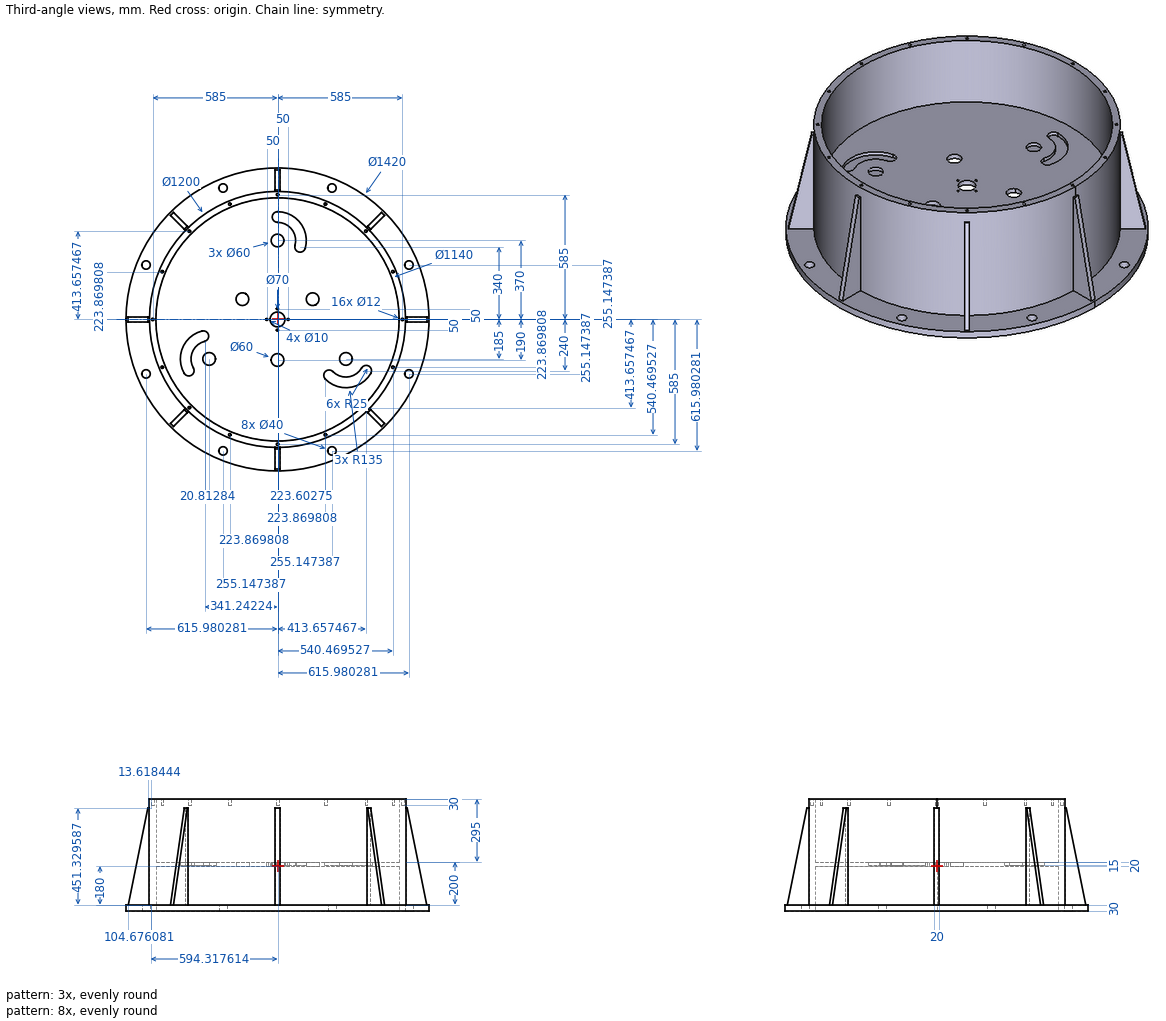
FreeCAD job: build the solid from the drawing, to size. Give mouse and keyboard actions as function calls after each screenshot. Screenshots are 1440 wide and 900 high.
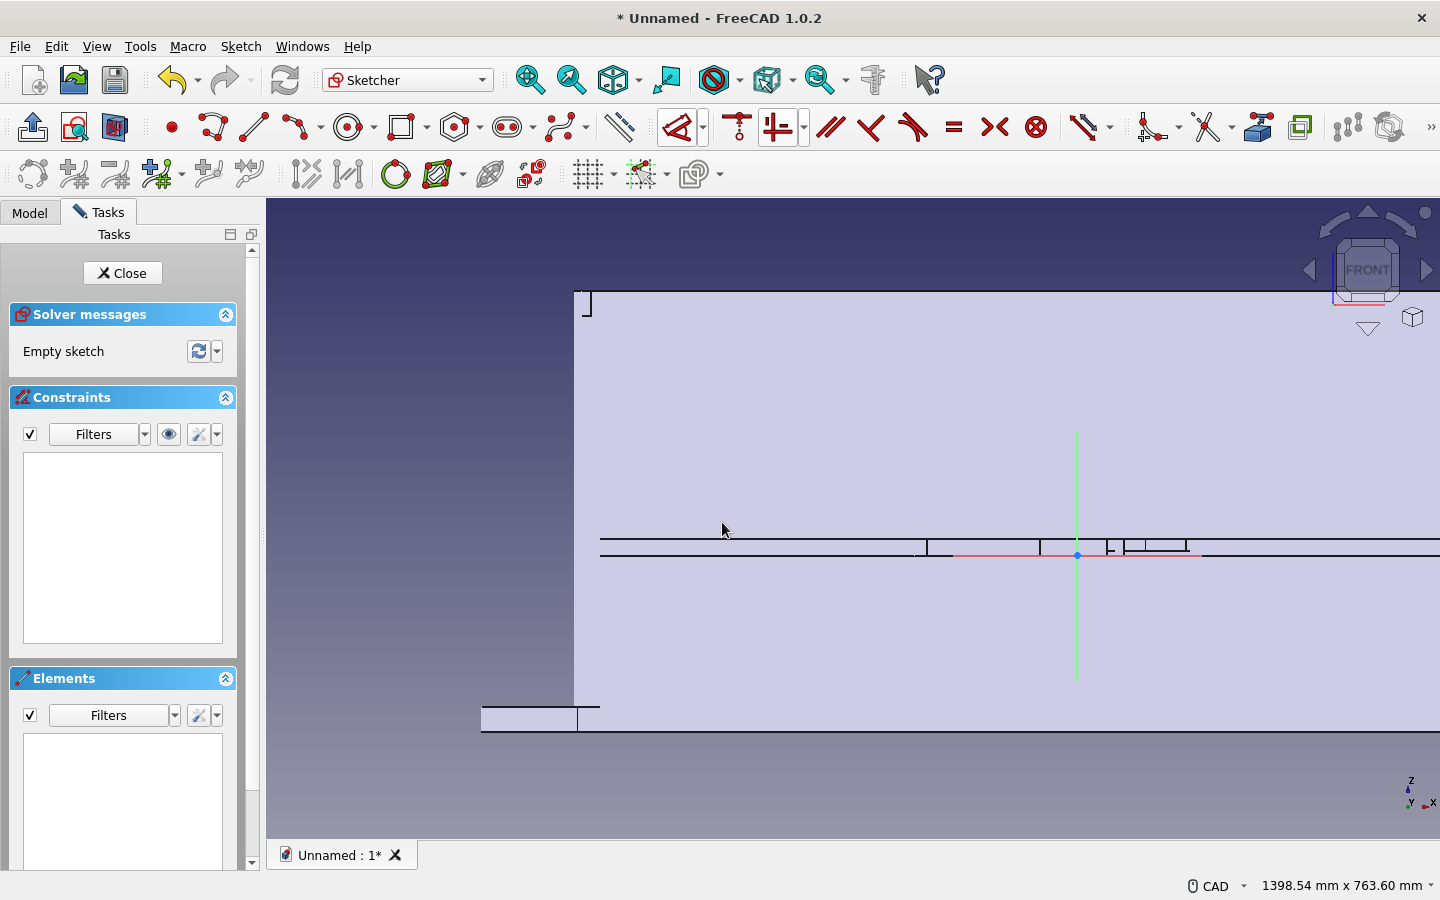
key(g)
key(m)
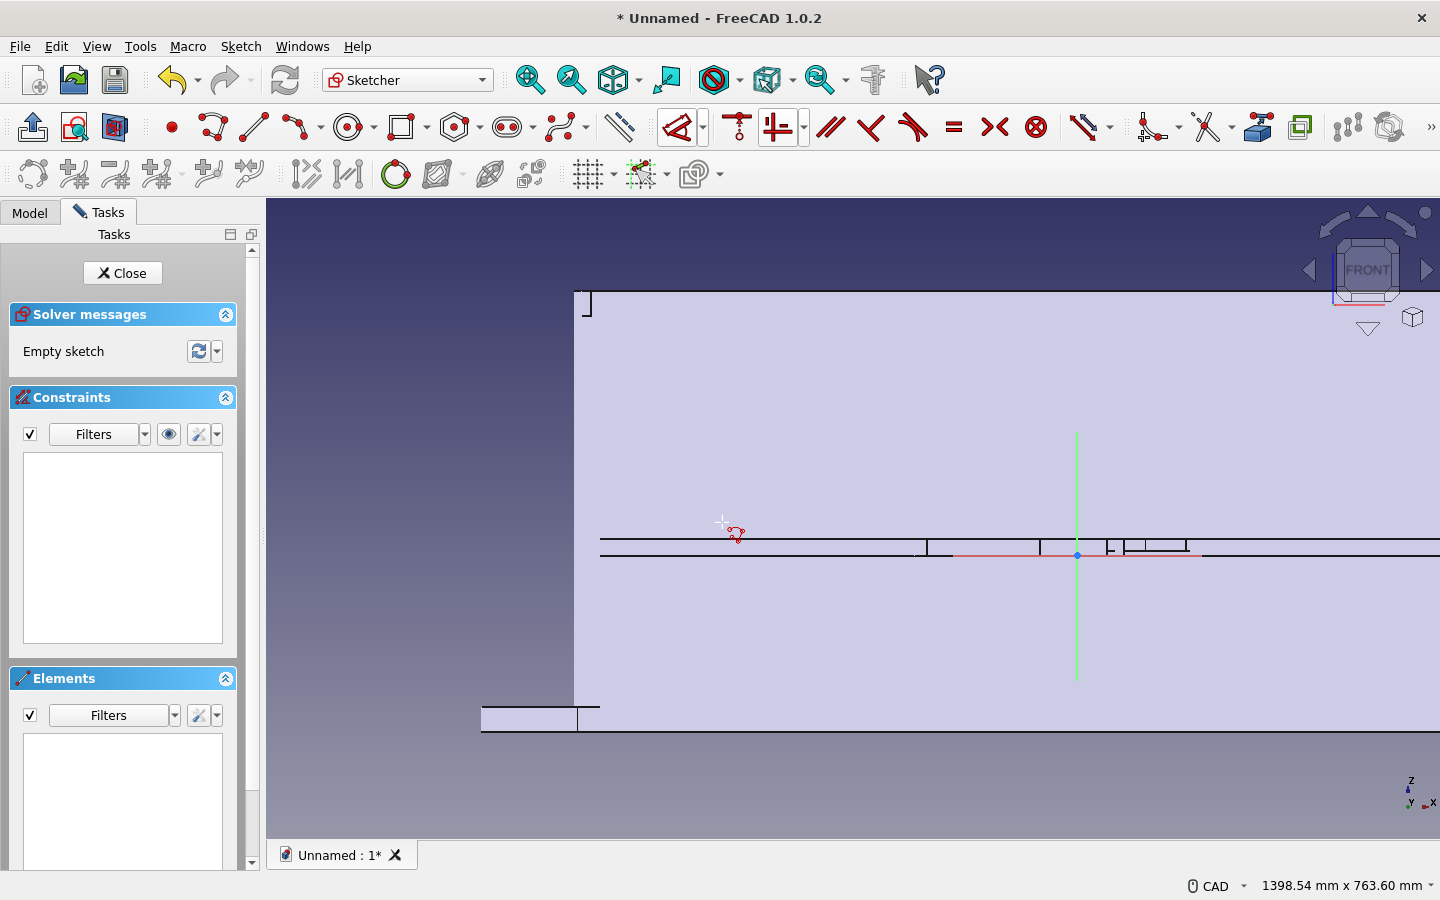
click(579, 707)
click(491, 707)
click(567, 328)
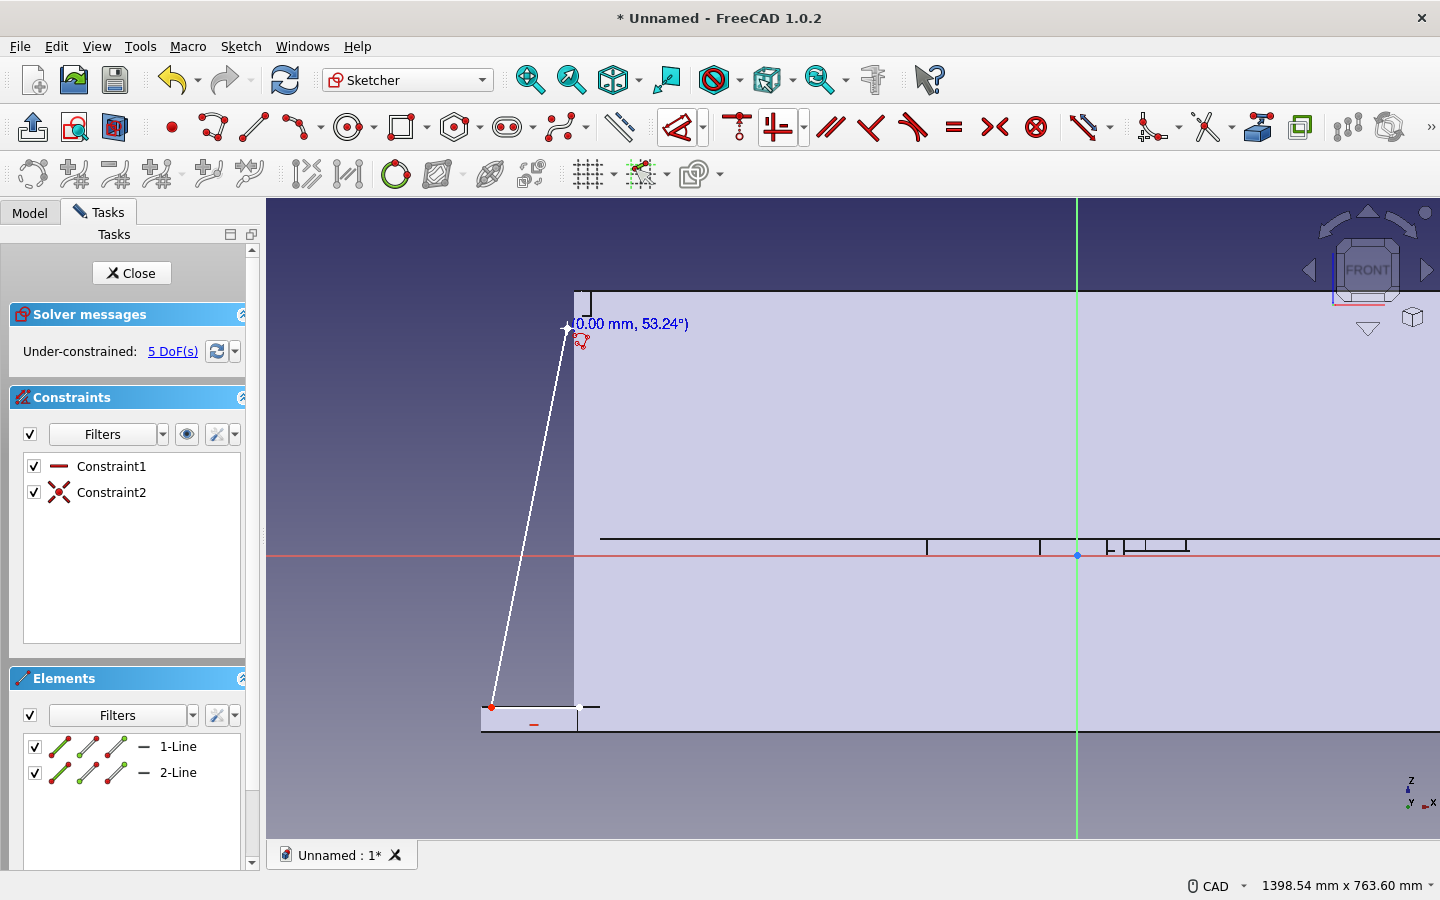
scroll(579, 328, up, 2)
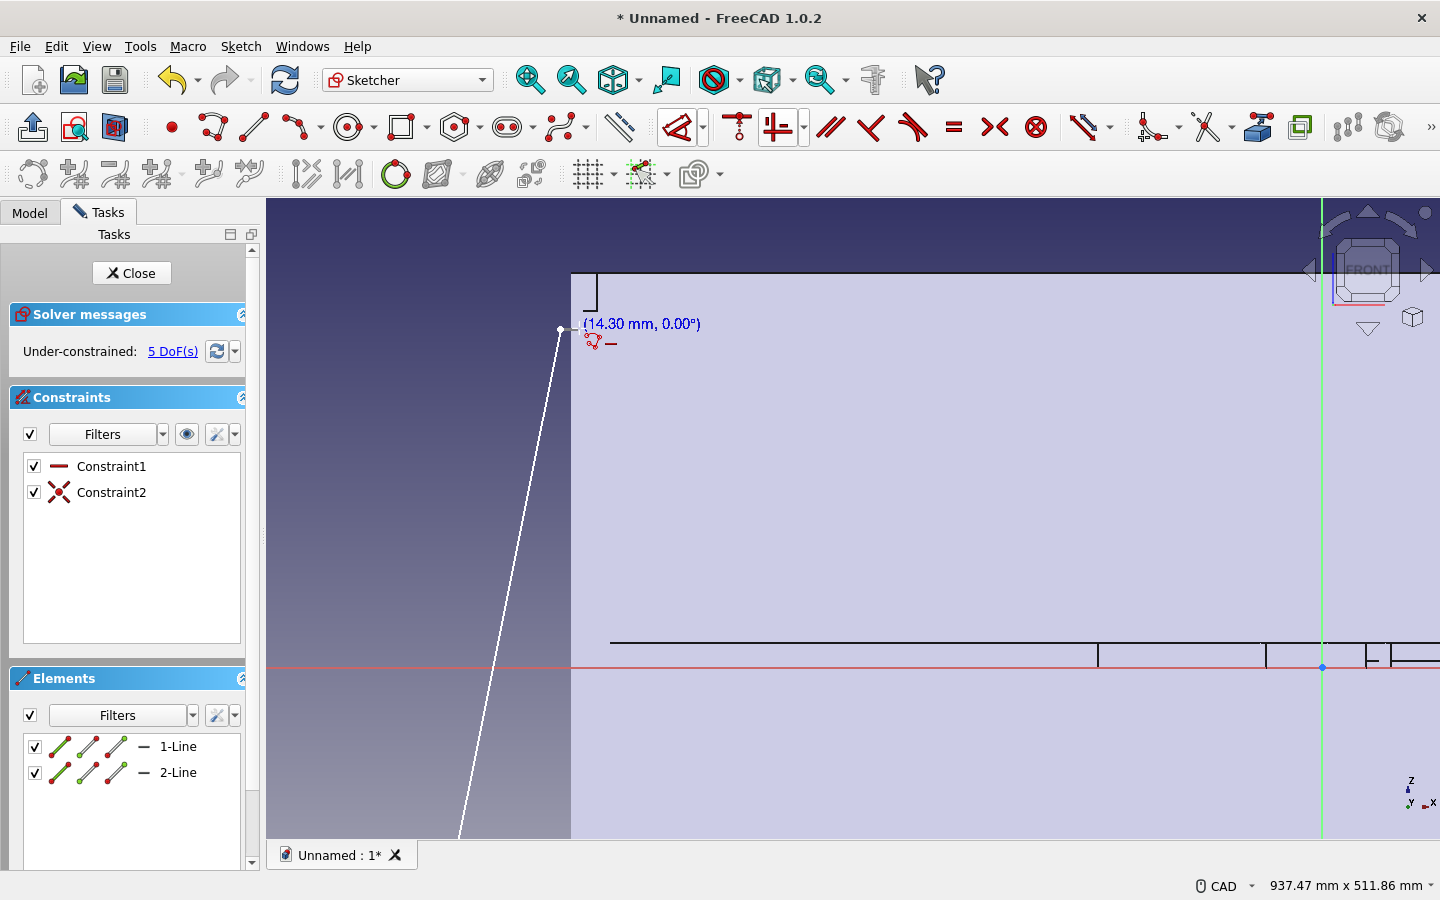
click(578, 328)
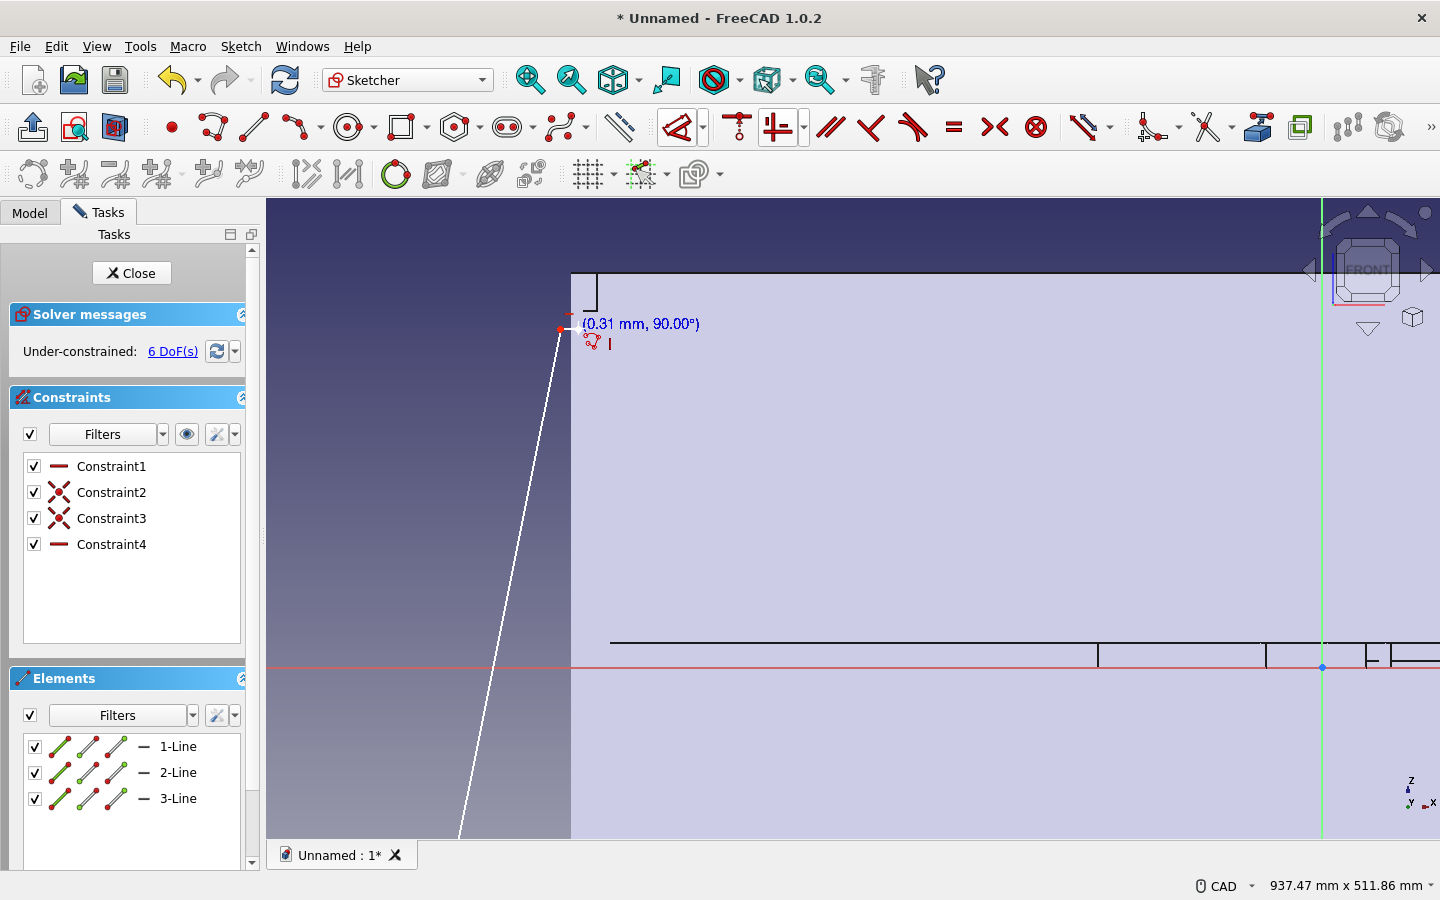
scroll(581, 332, down, 2)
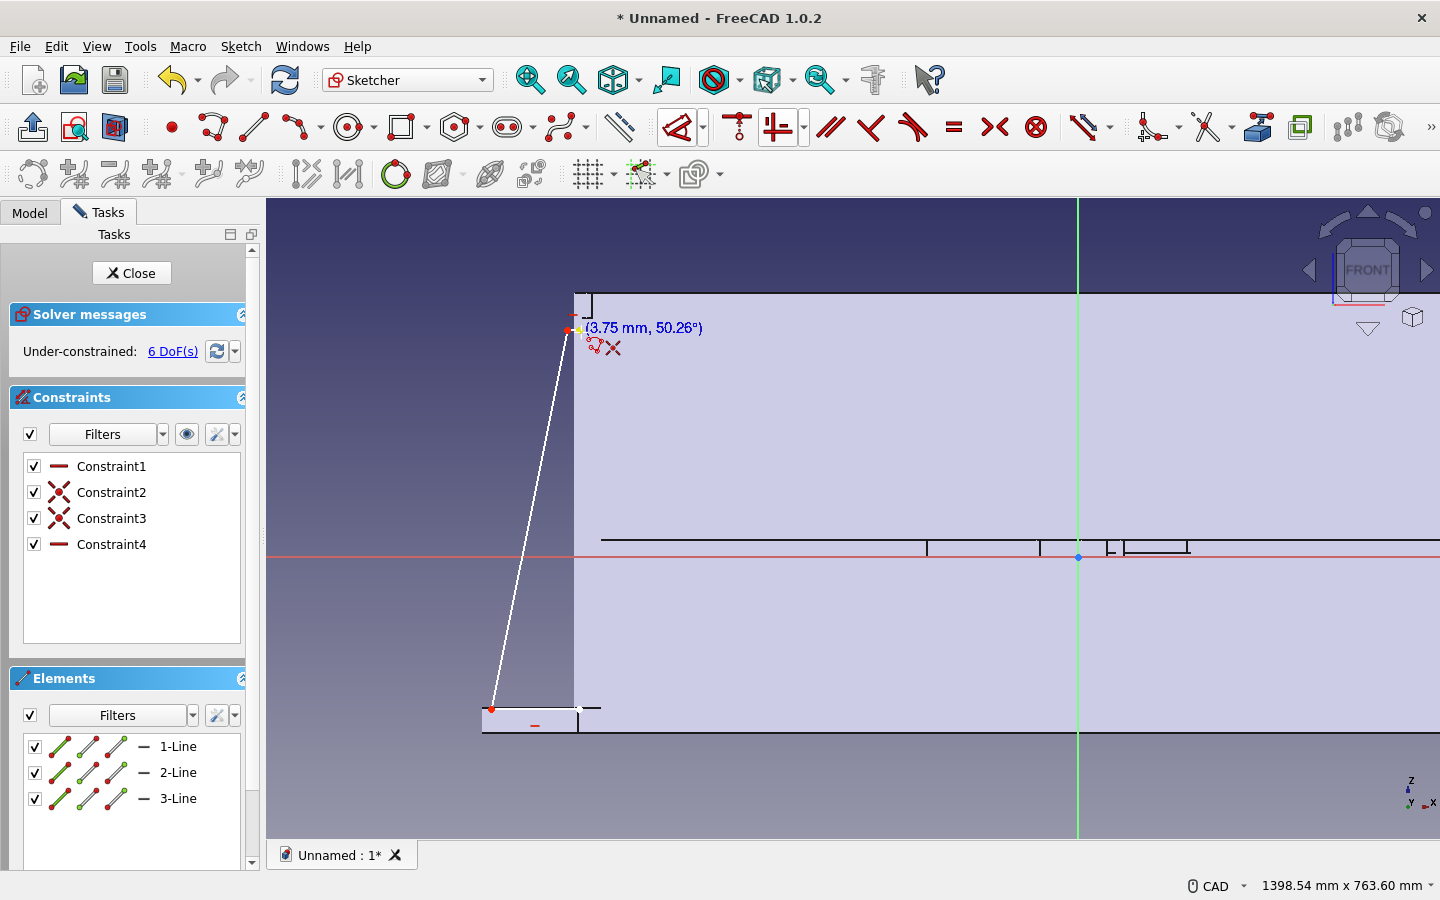
click(580, 709)
key(Escape)
key(Escape)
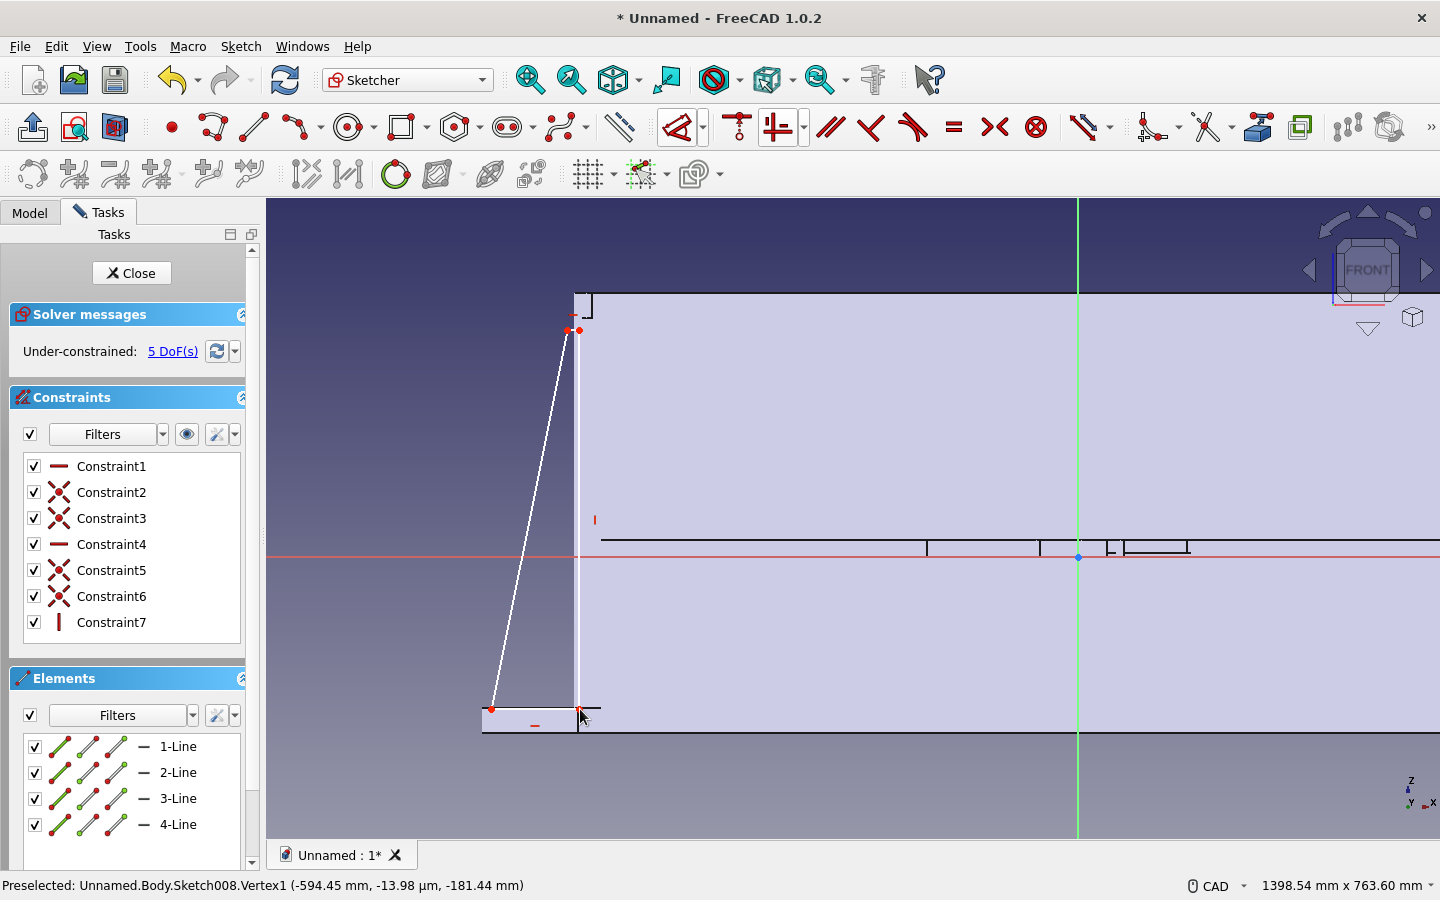
click(579, 709)